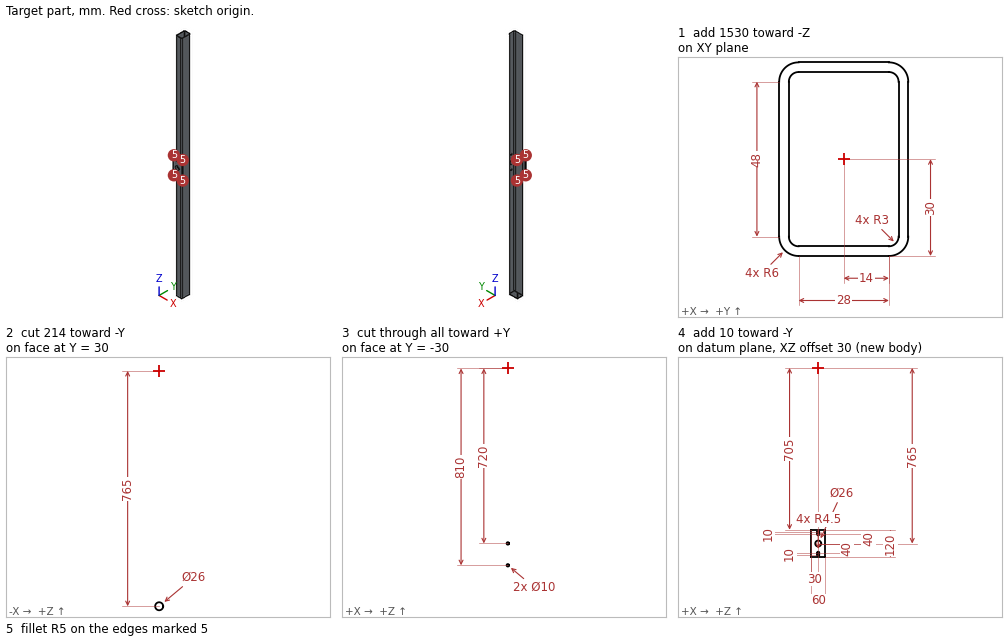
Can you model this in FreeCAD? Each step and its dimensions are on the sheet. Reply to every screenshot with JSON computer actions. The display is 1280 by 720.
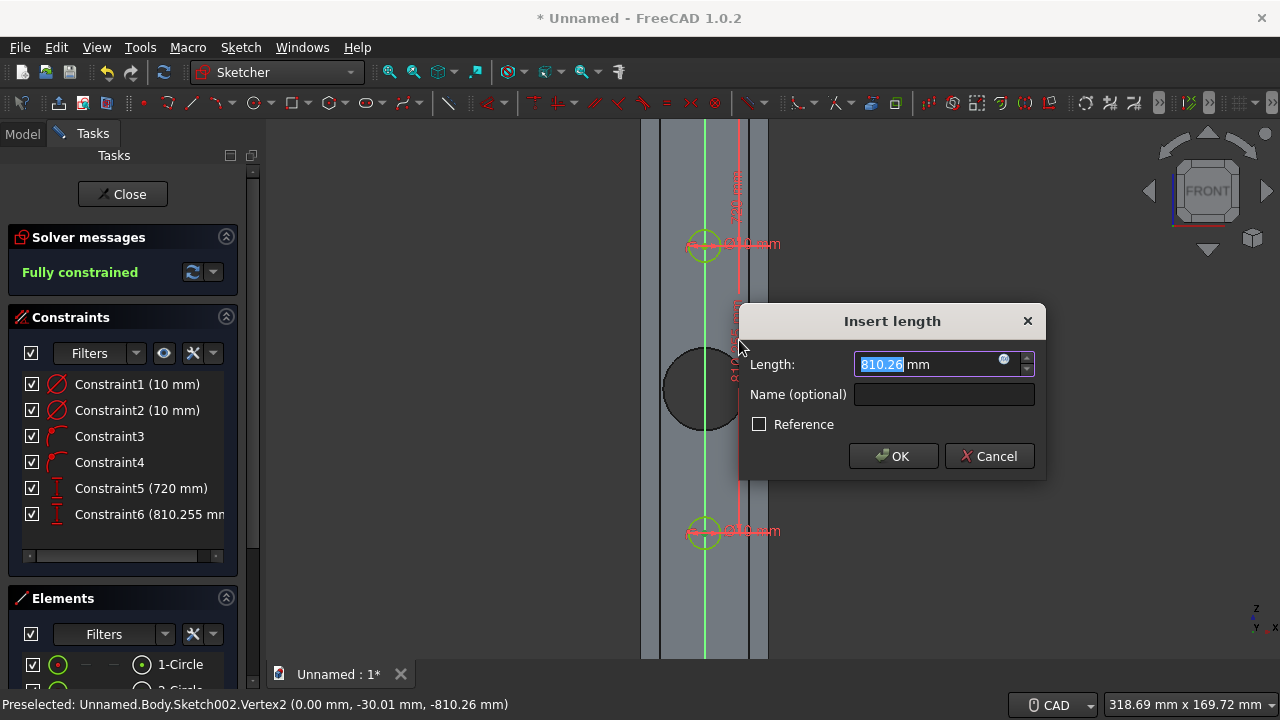
{"action": "type", "text": "810"}
{"action": "key", "text": "Return"}
{"action": "key", "text": "Escape"}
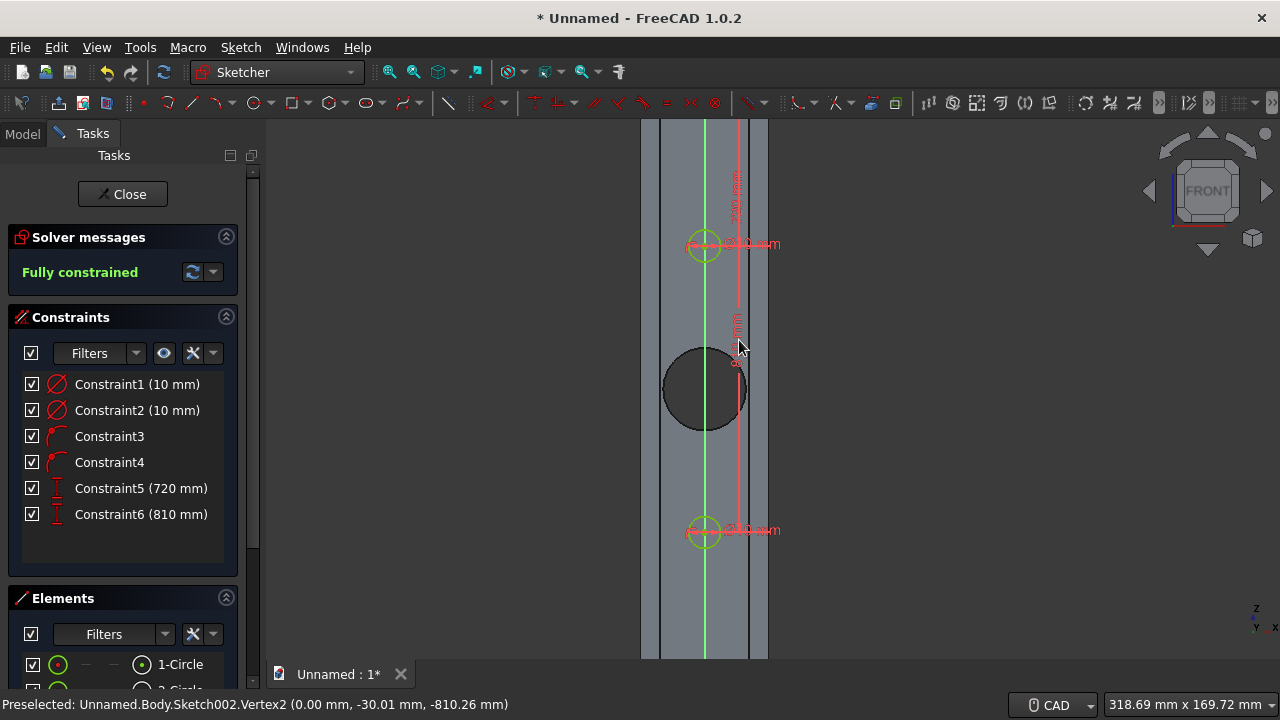
{"action": "left_click", "coordinate": [123, 194]}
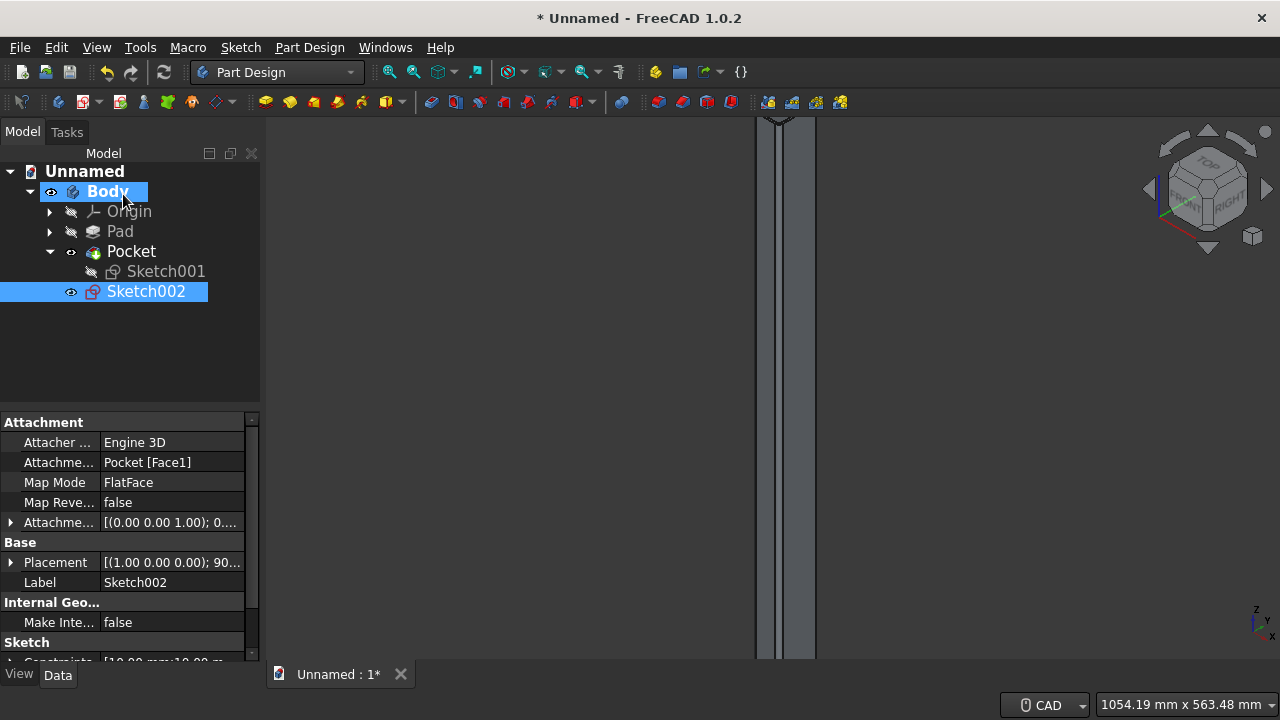
{"action": "left_click", "coordinate": [432, 102]}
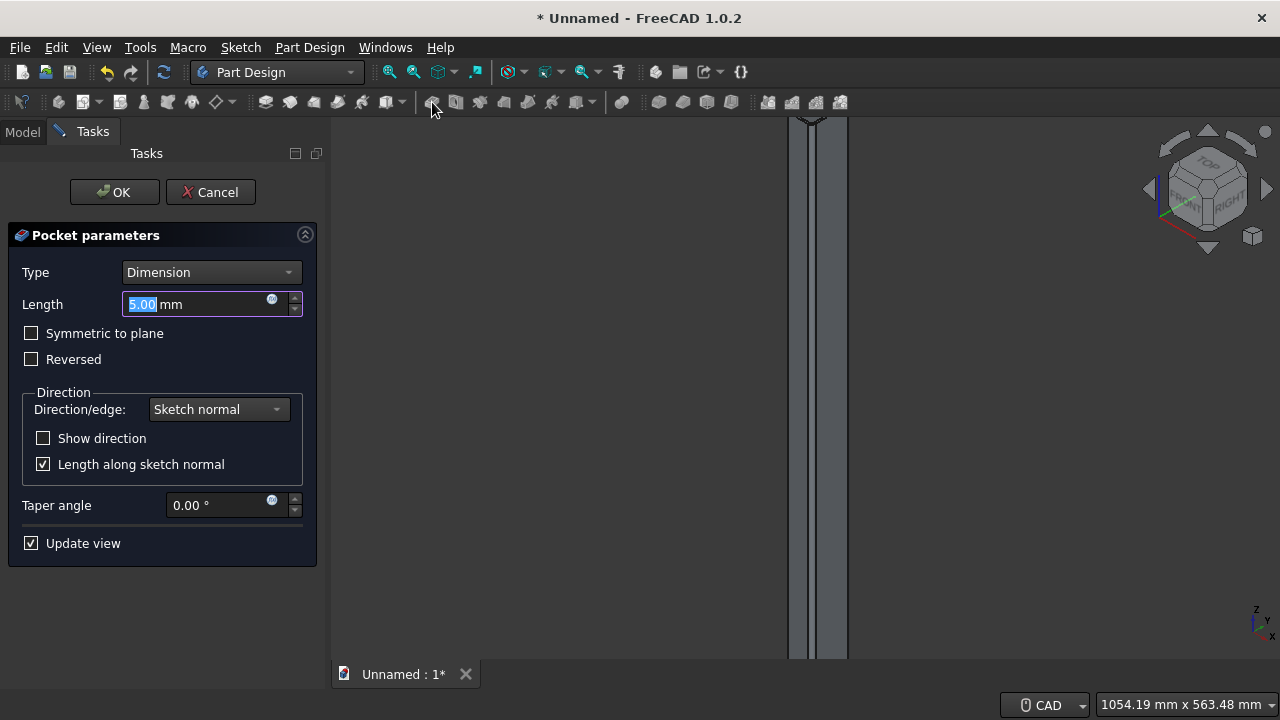
{"action": "left_click", "coordinate": [212, 272]}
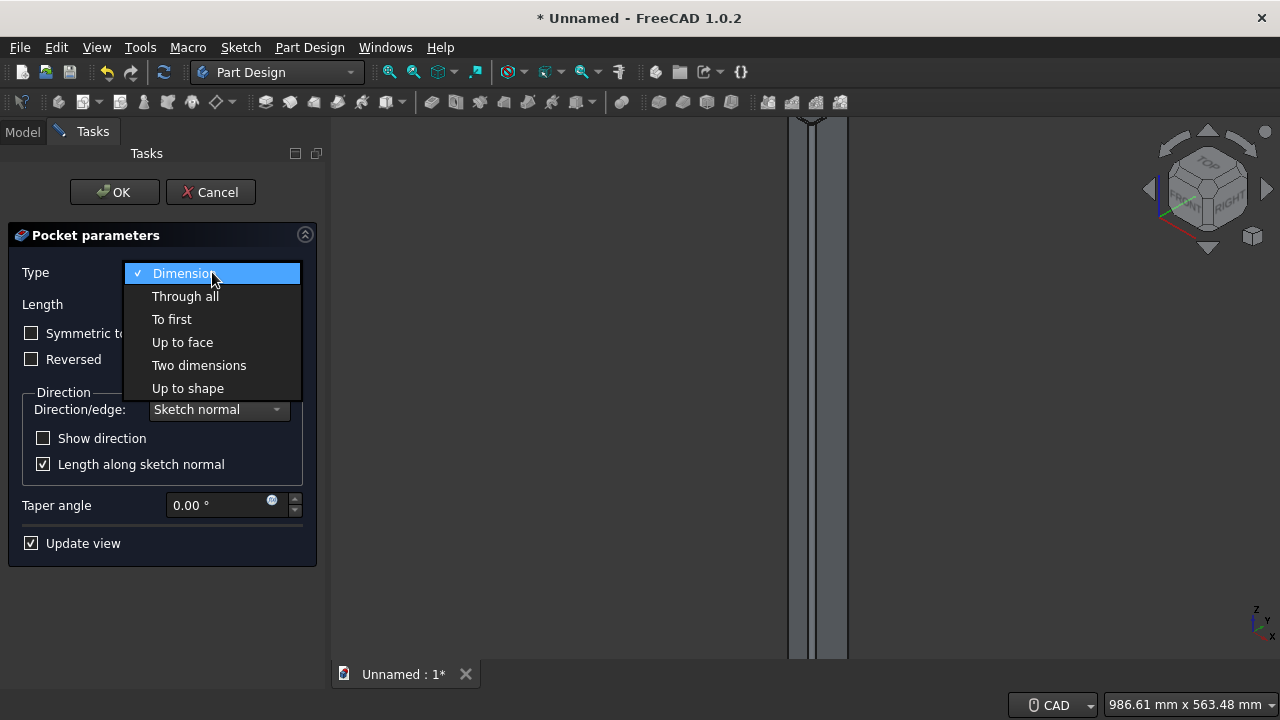
{"action": "left_click", "coordinate": [212, 296]}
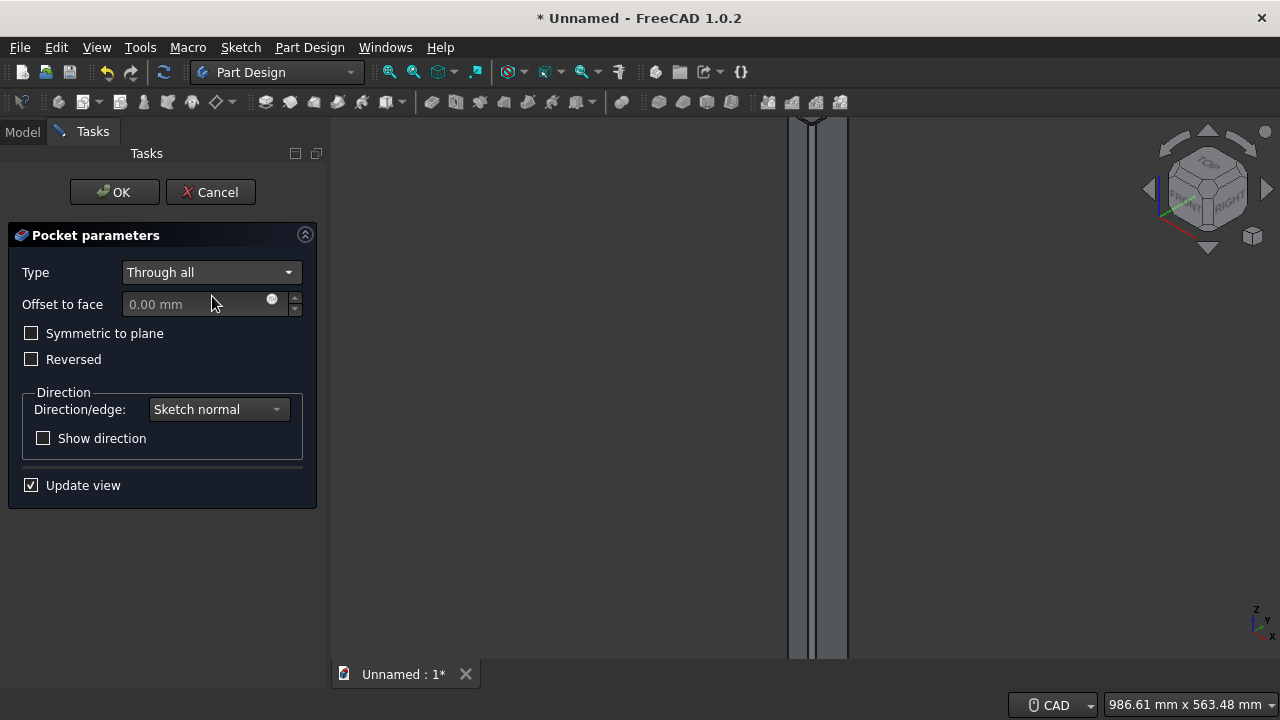
{"action": "left_click", "coordinate": [115, 192]}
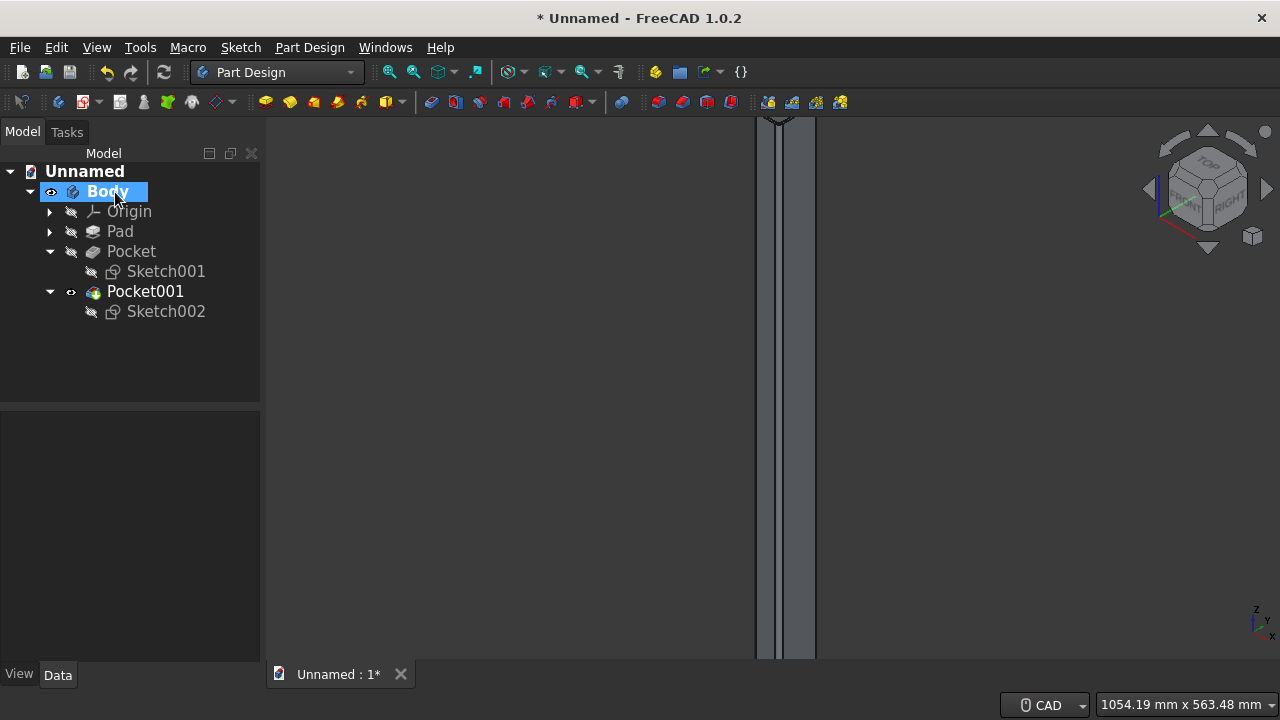
{"action": "left_click", "coordinate": [390, 72]}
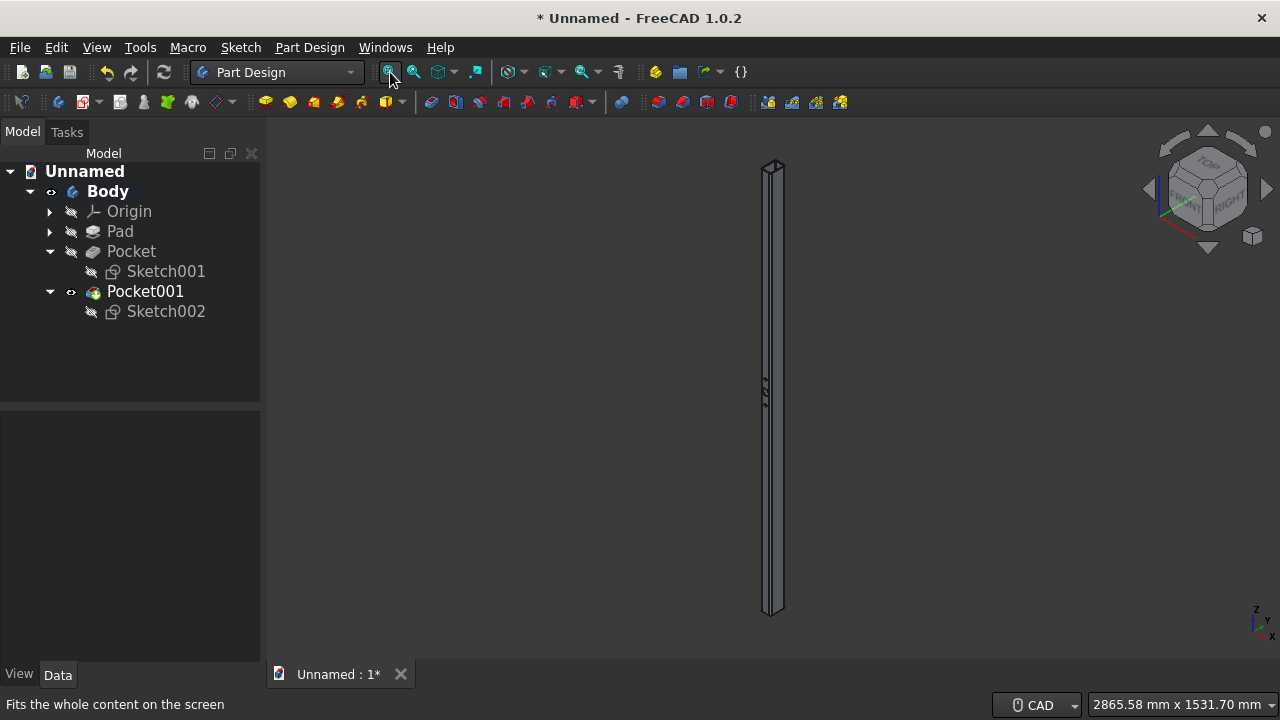
{"action": "left_click", "coordinate": [60, 102]}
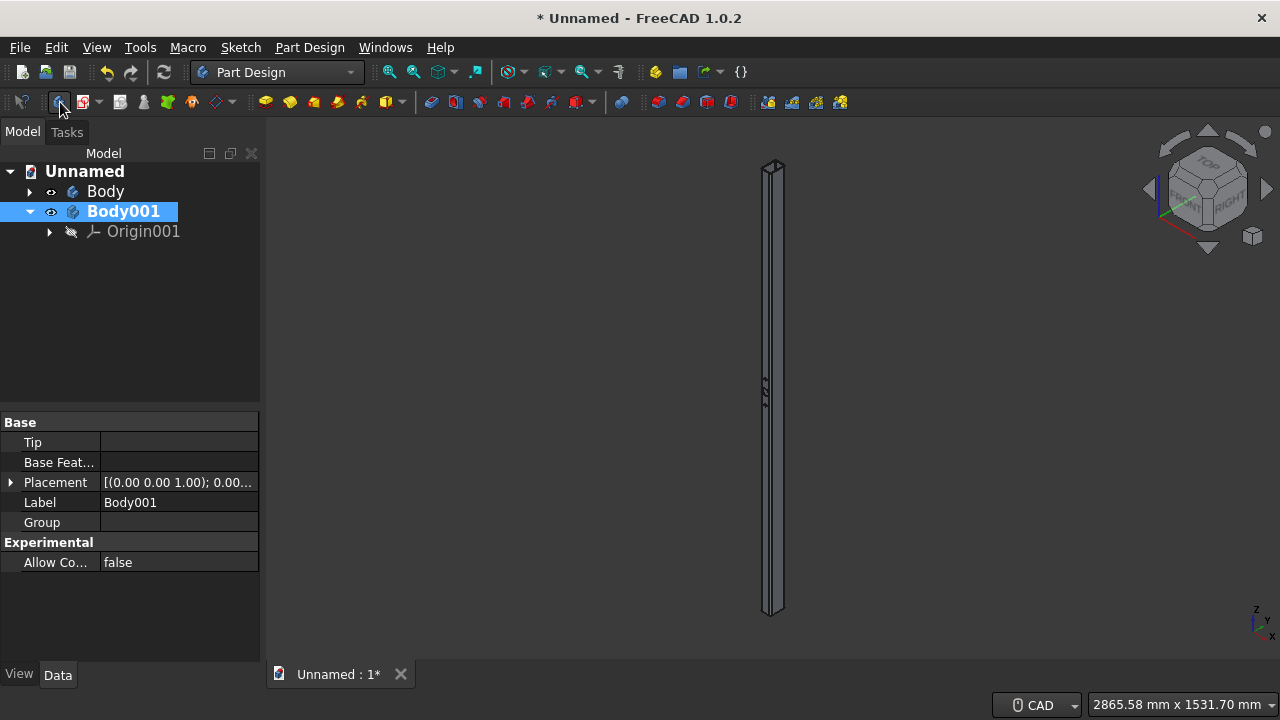
{"action": "left_click", "coordinate": [50, 232]}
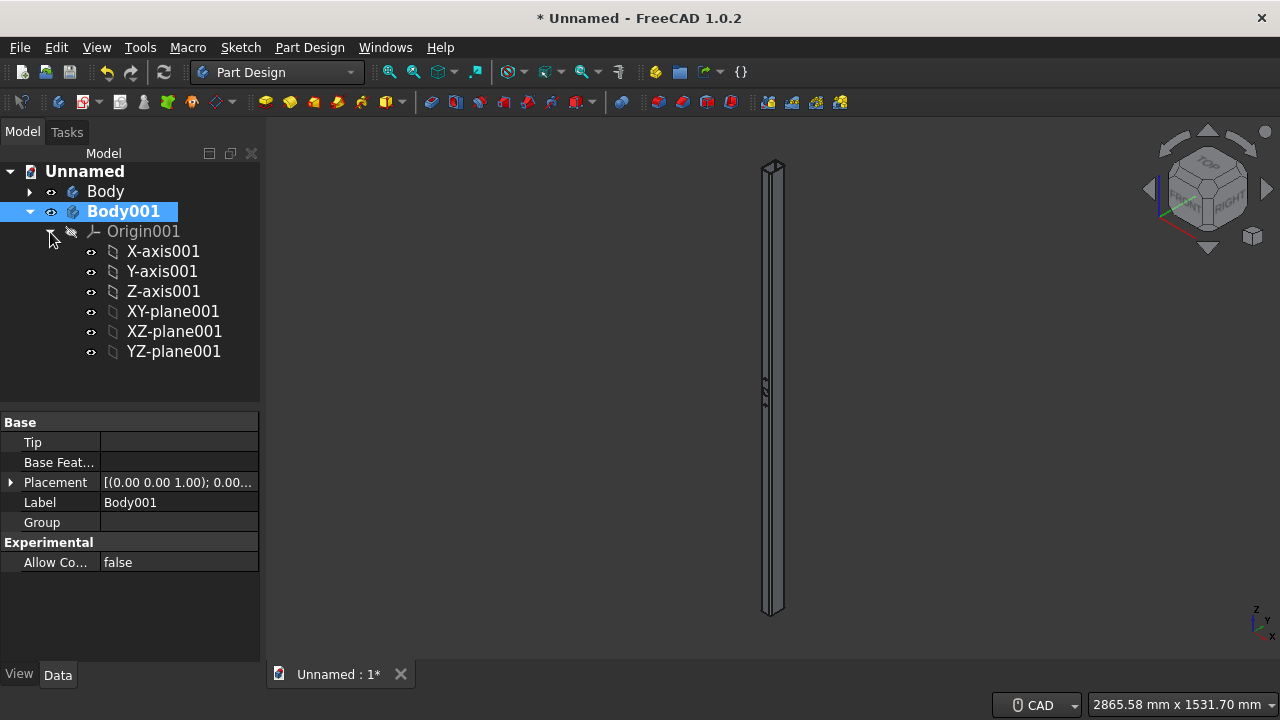
{"action": "left_click", "coordinate": [136, 332]}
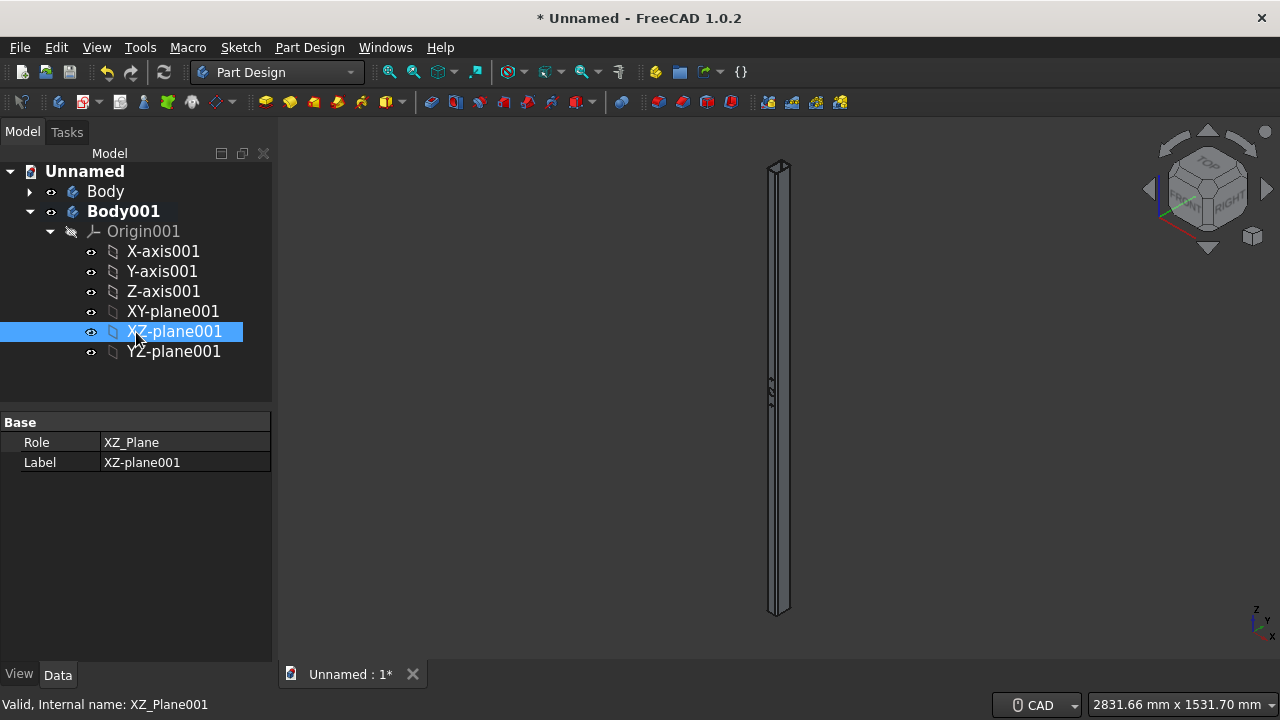
{"action": "left_click", "coordinate": [216, 102]}